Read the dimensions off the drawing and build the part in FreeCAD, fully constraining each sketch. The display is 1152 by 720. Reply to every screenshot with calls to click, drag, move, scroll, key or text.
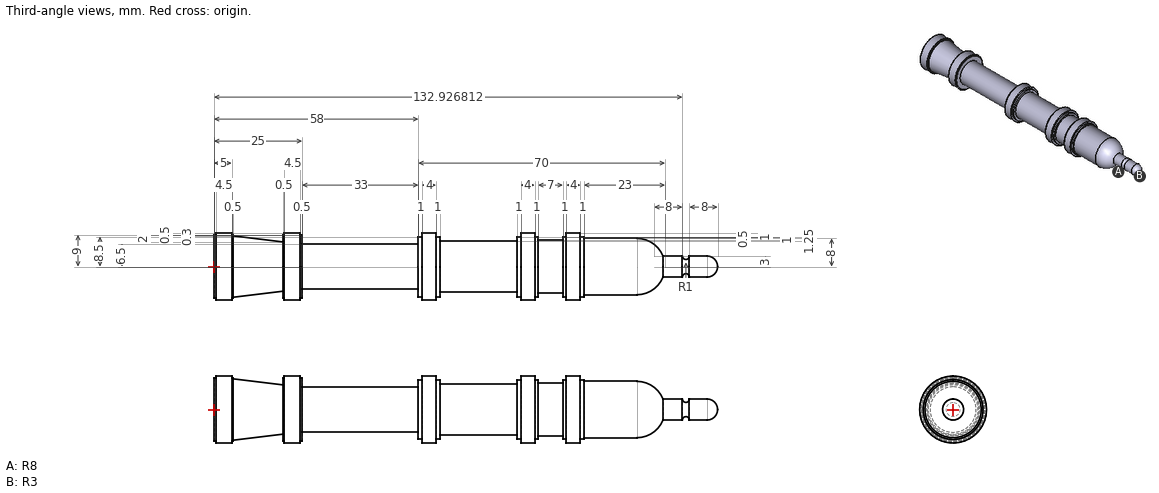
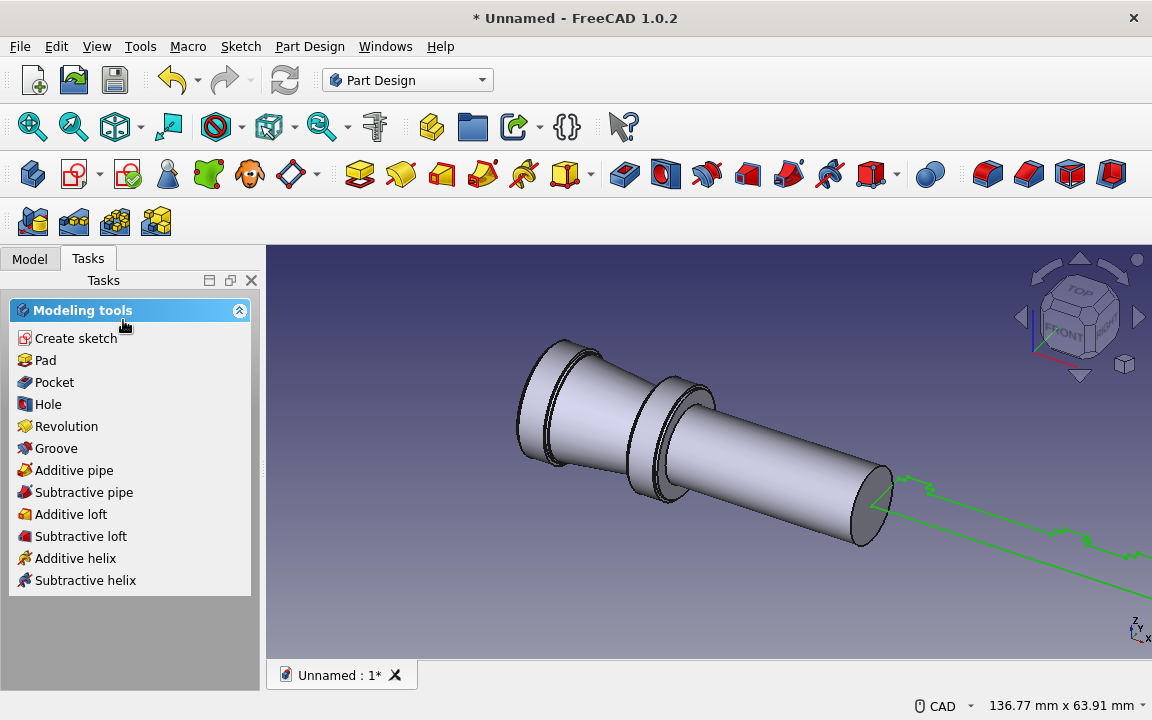
click(401, 174)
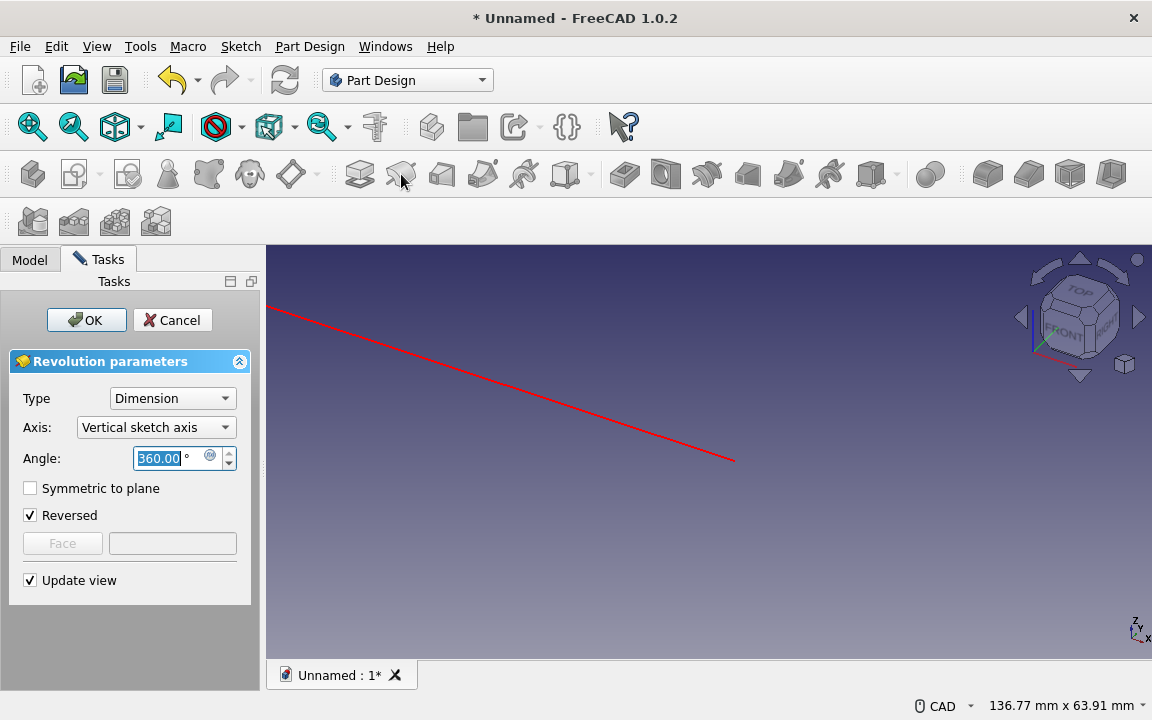
click(157, 428)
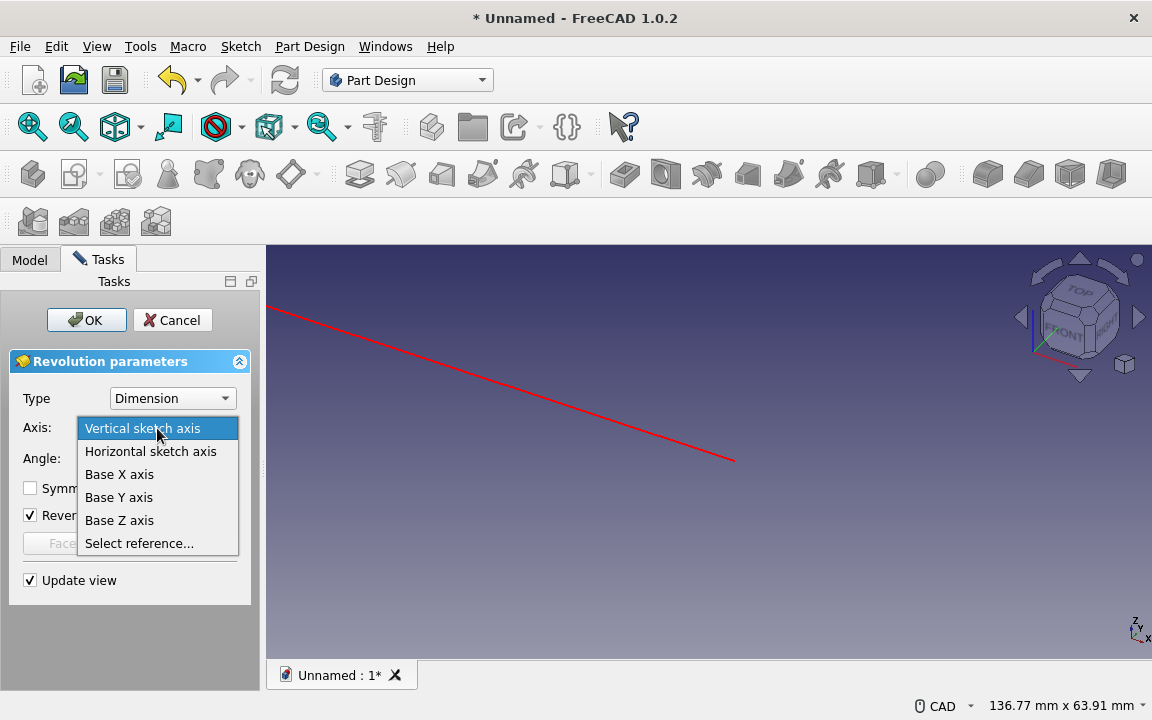
click(156, 452)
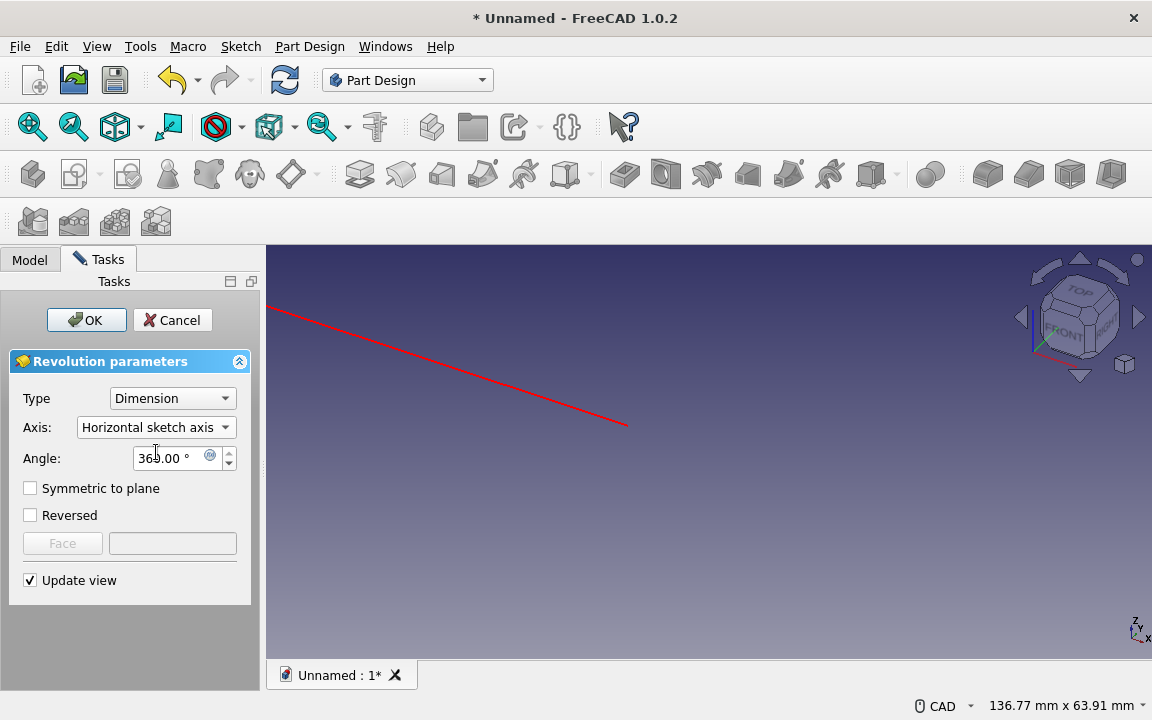
click(87, 320)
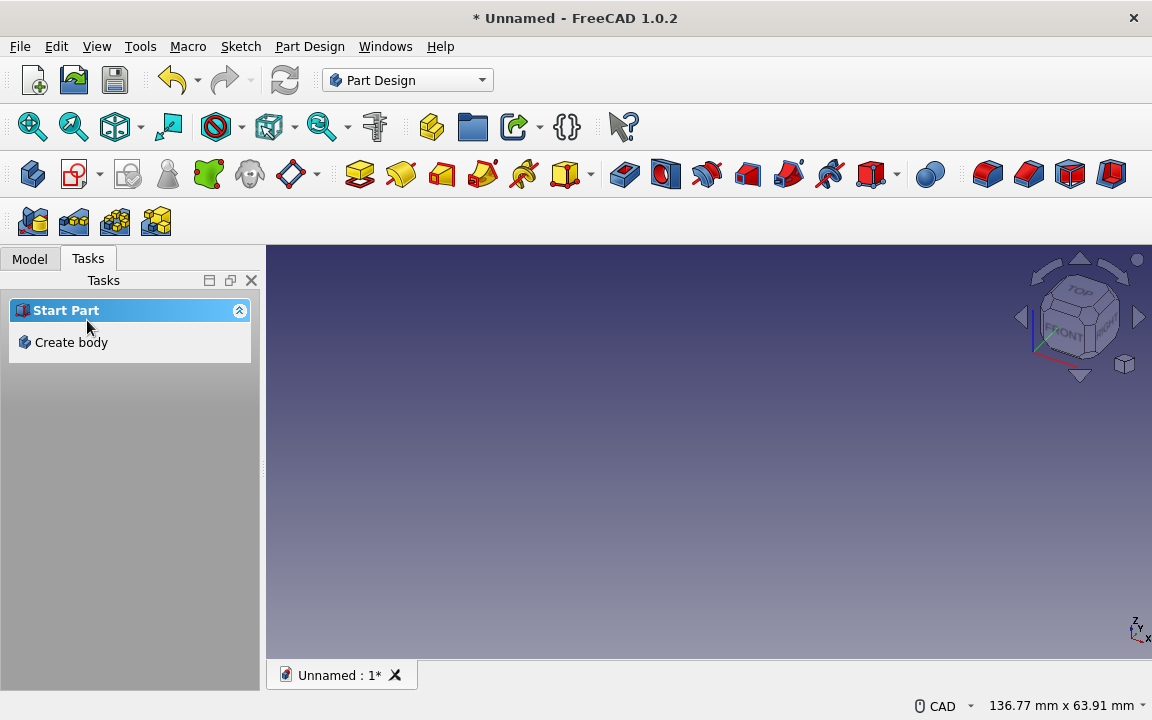
click(33, 128)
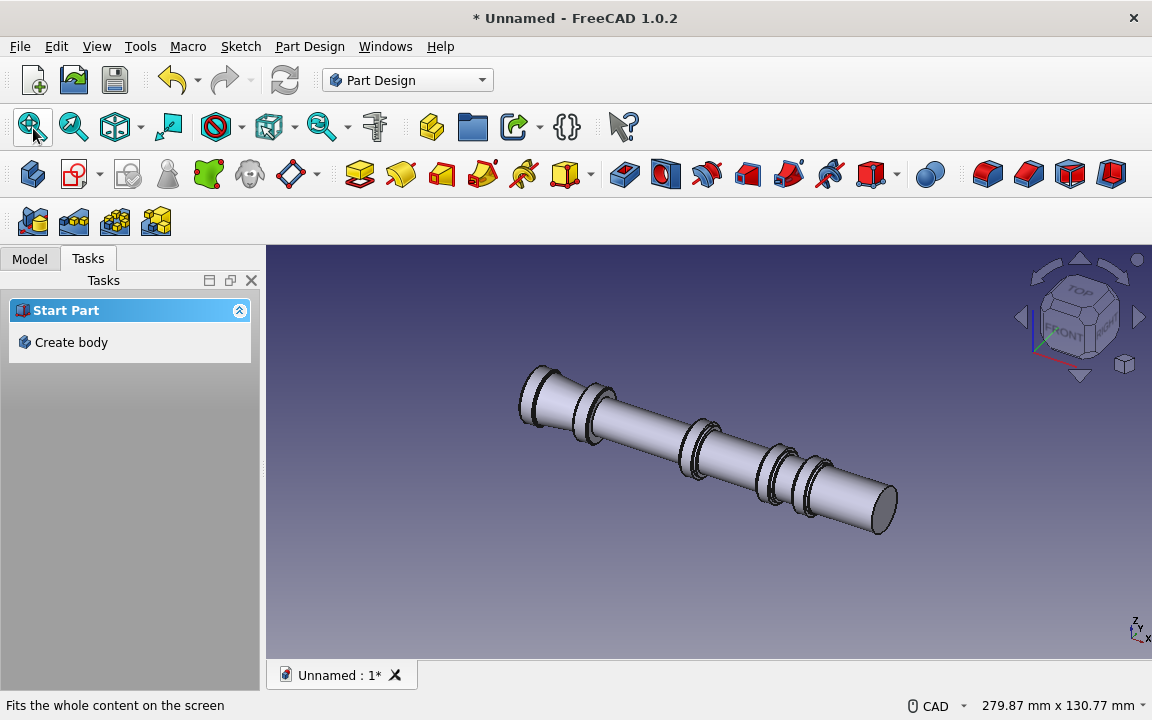
click(872, 522)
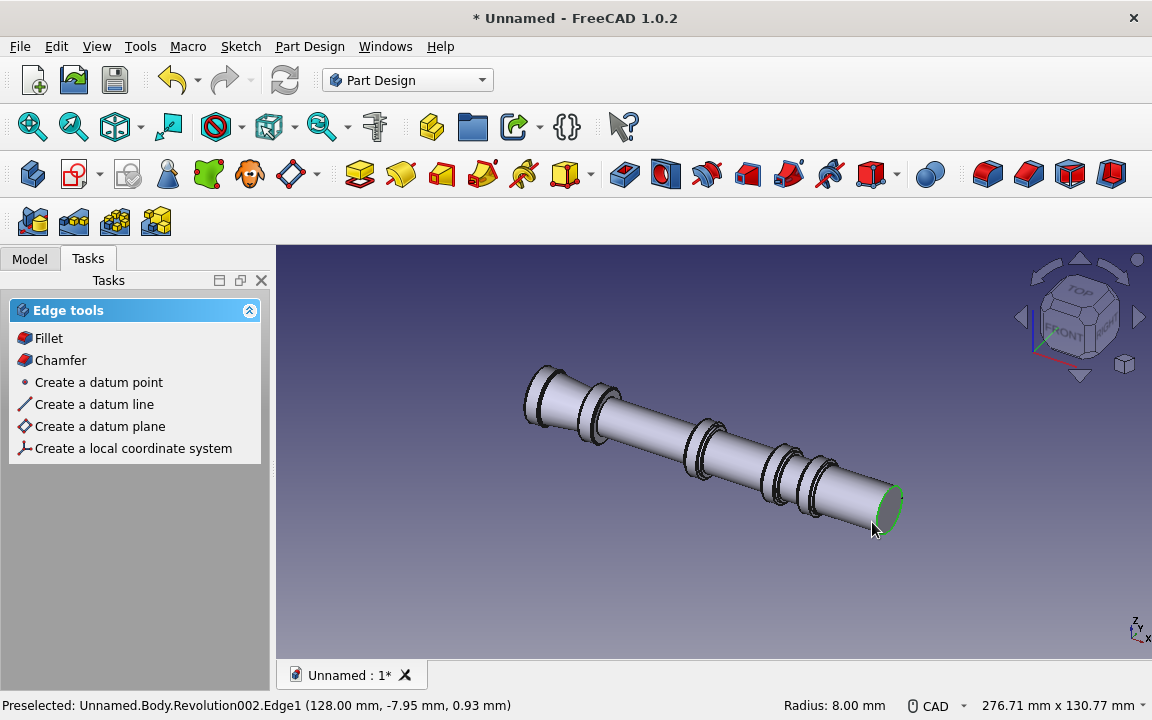
click(988, 174)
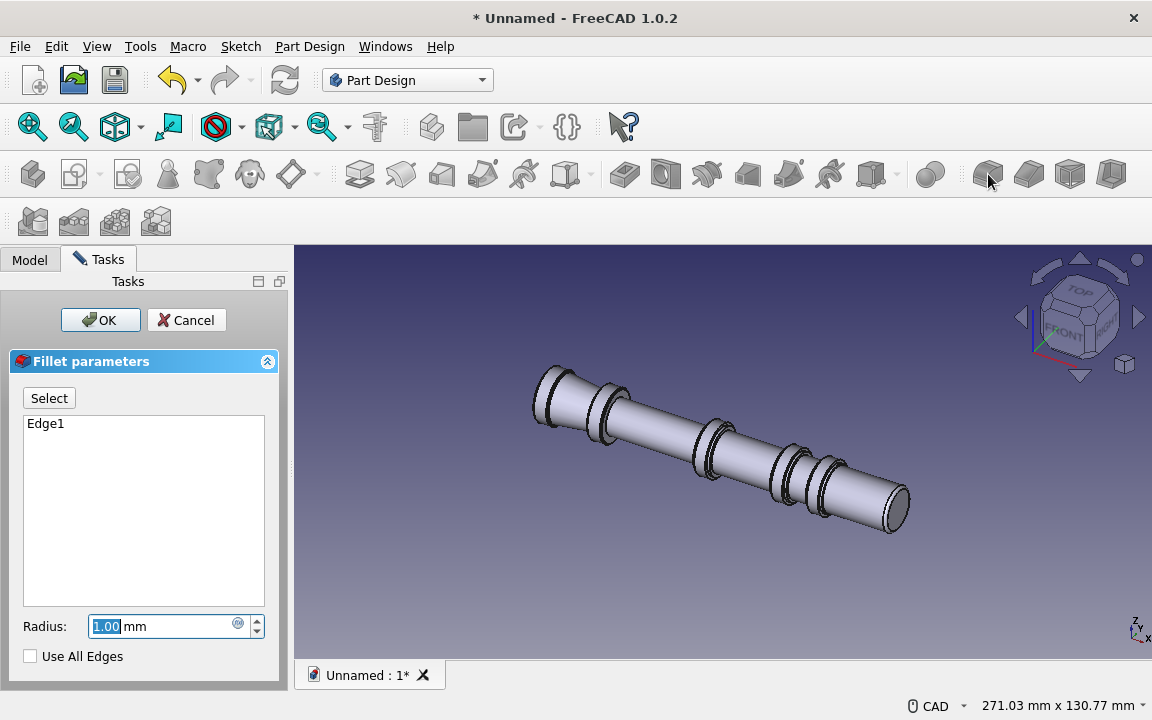
text(8)
key(Tab)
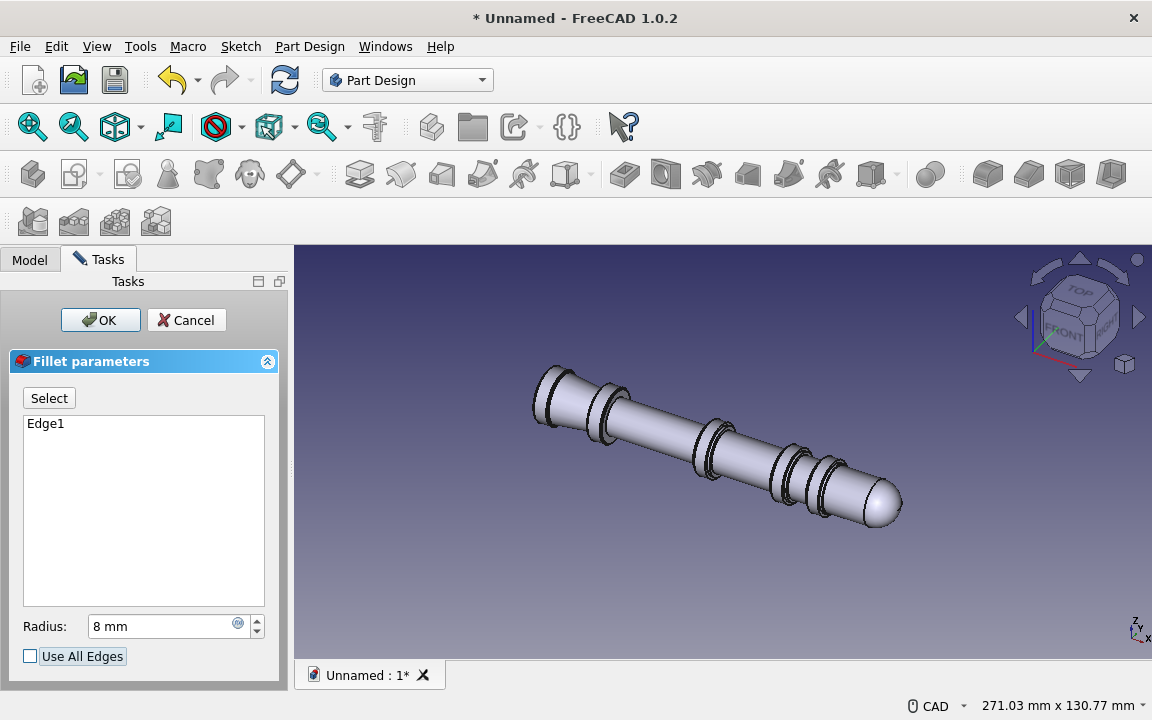
click(101, 320)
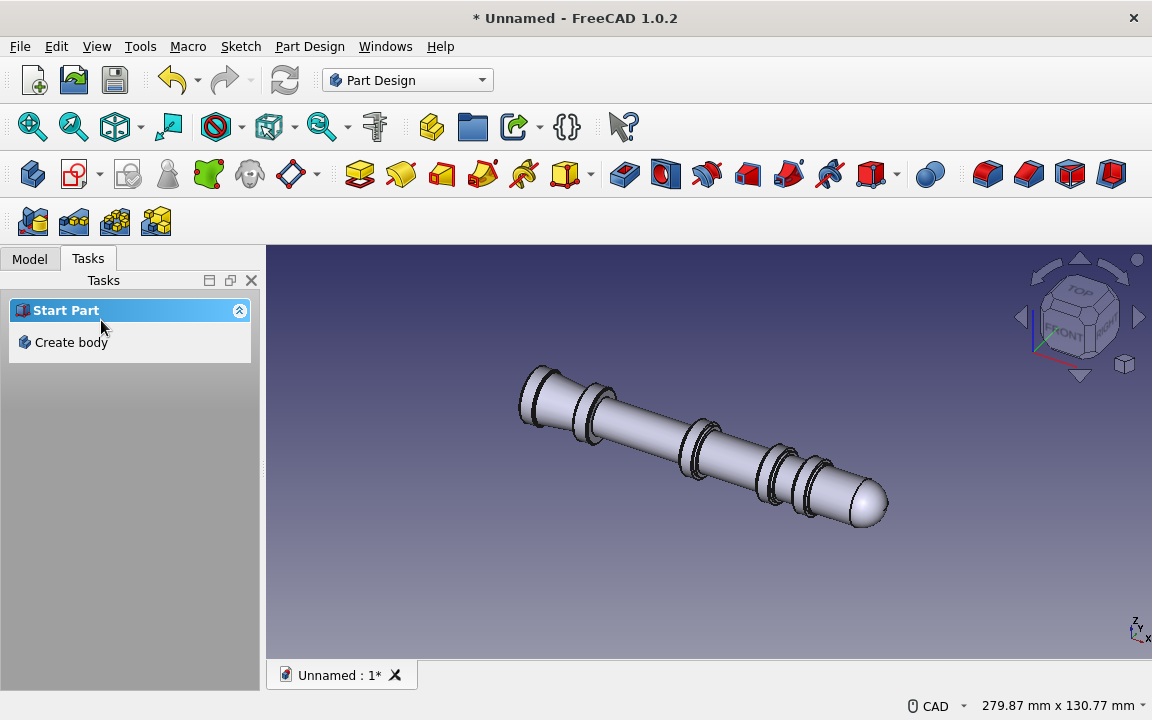
click(74, 174)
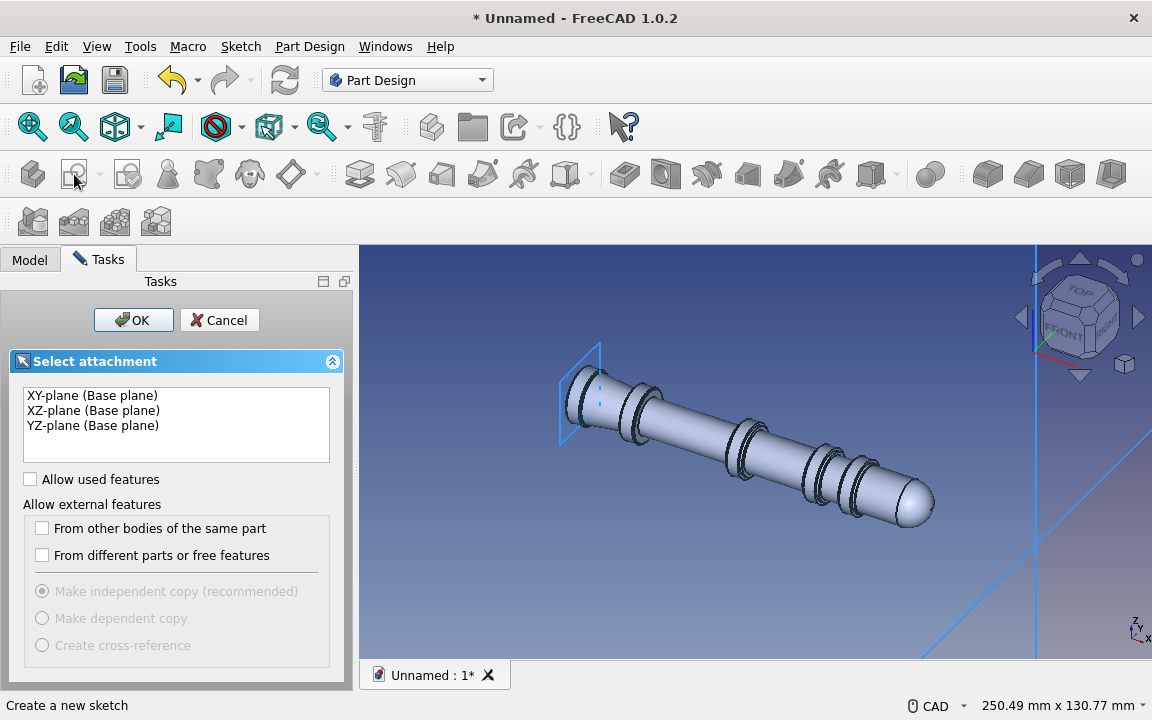
click(84, 396)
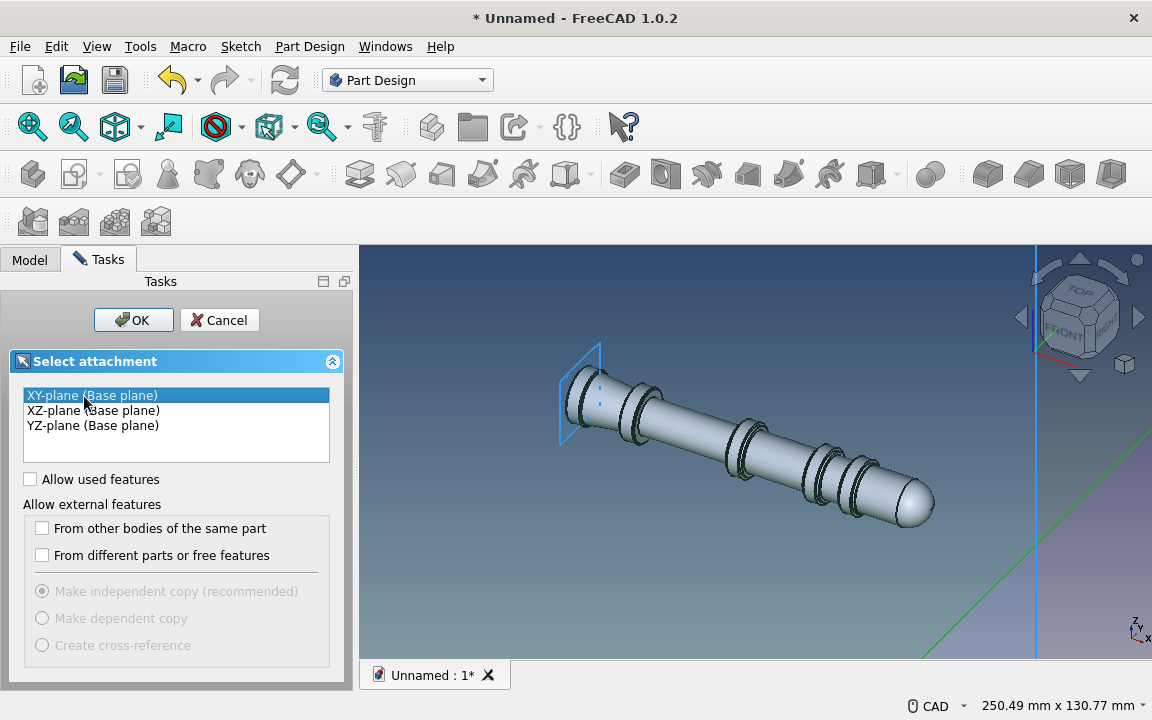
click(134, 320)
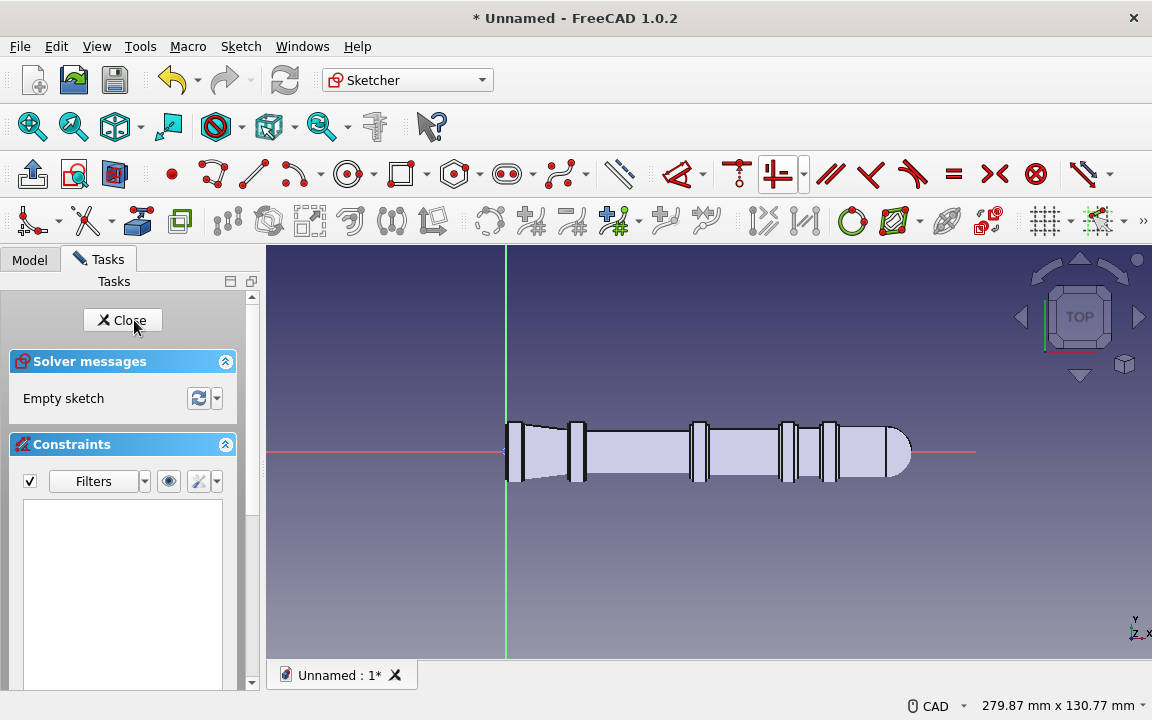
click(115, 174)